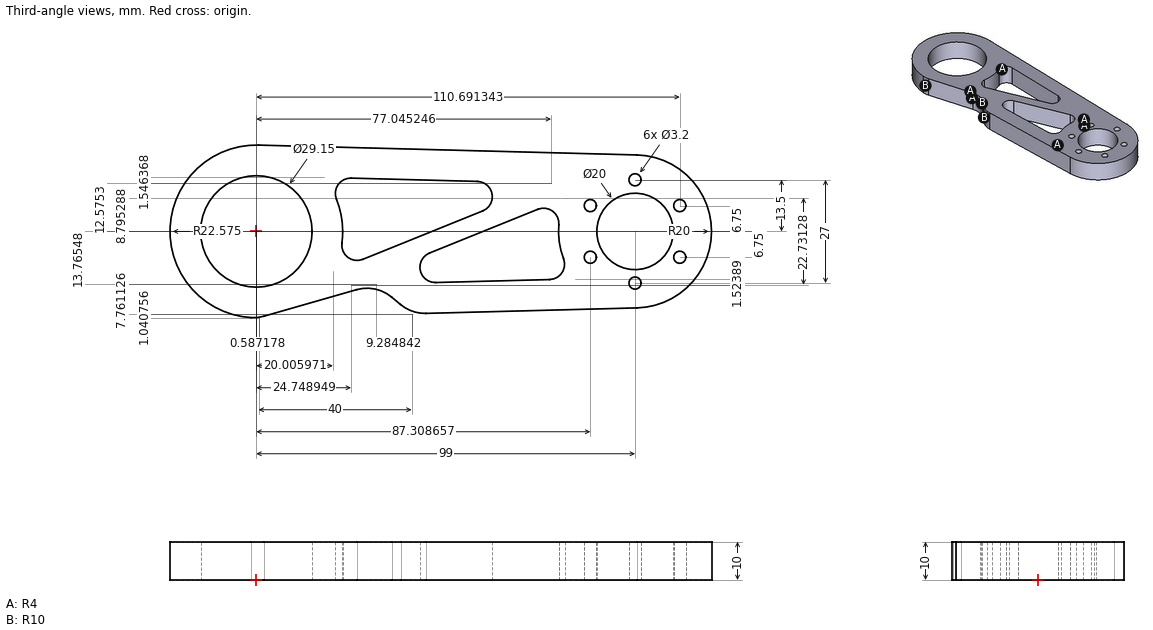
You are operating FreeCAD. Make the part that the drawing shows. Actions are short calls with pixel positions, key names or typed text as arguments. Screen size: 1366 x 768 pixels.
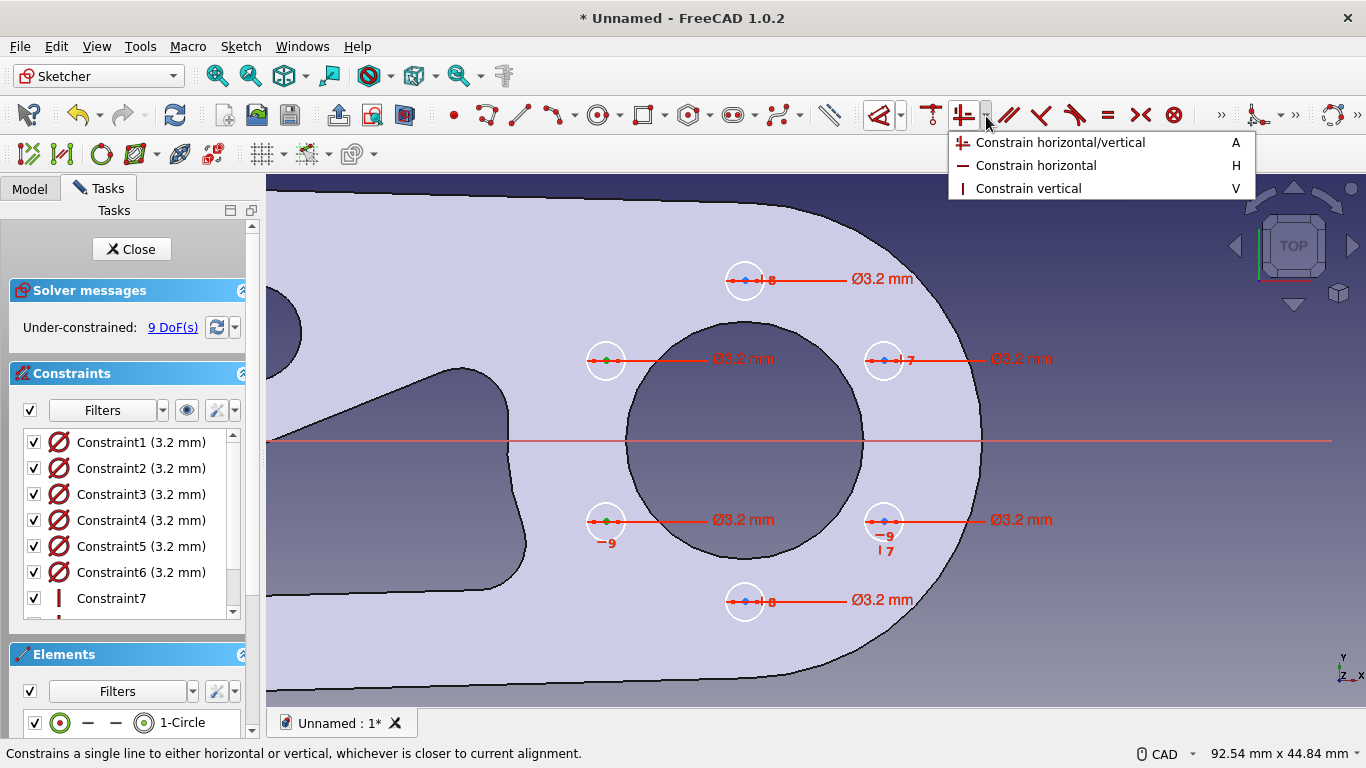
click(1102, 188)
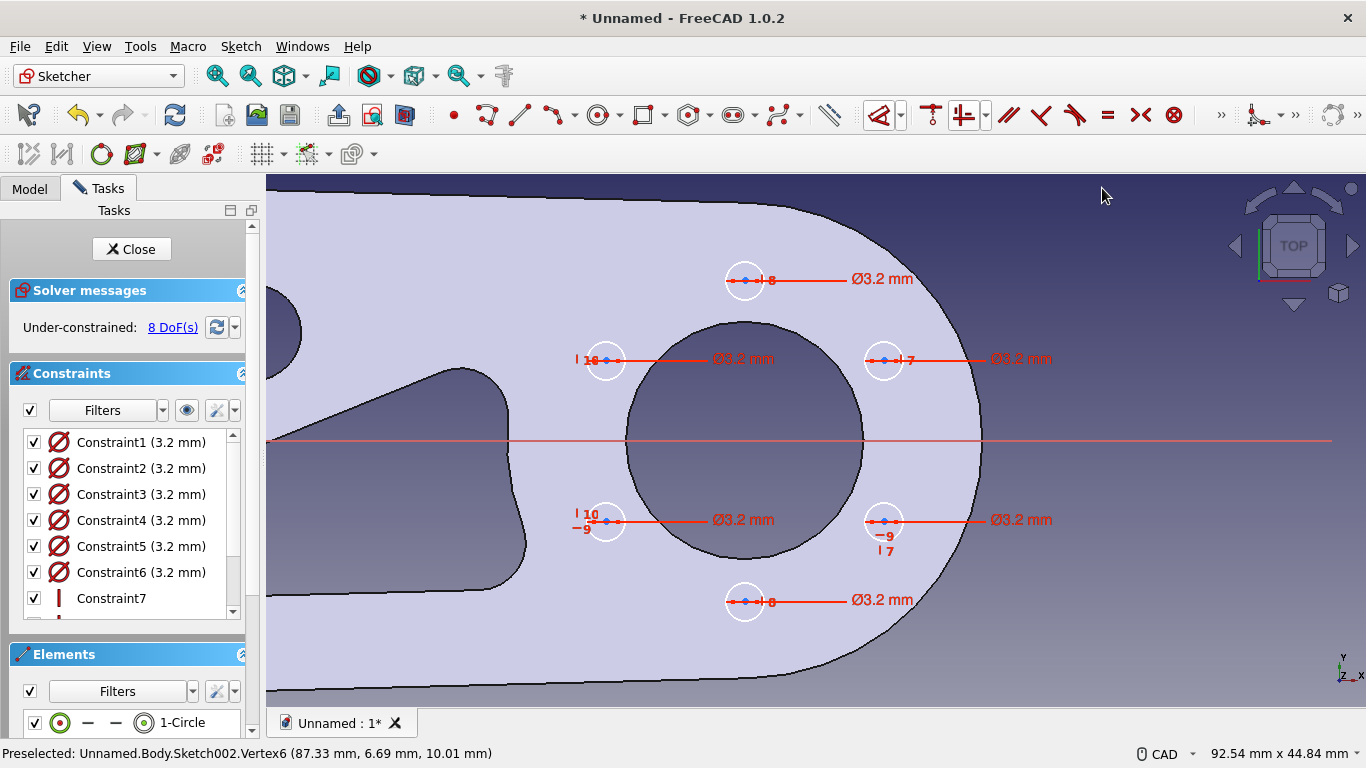
click(884, 361)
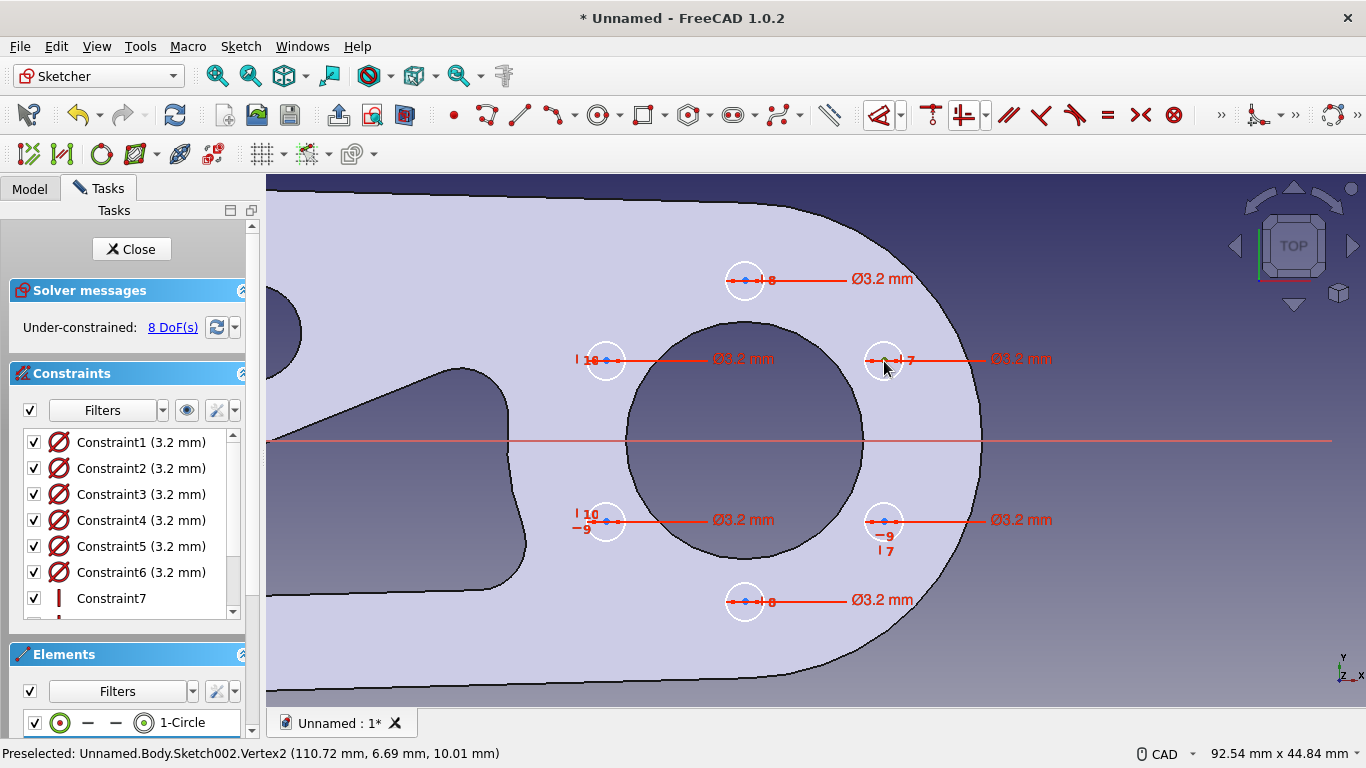
click(606, 361)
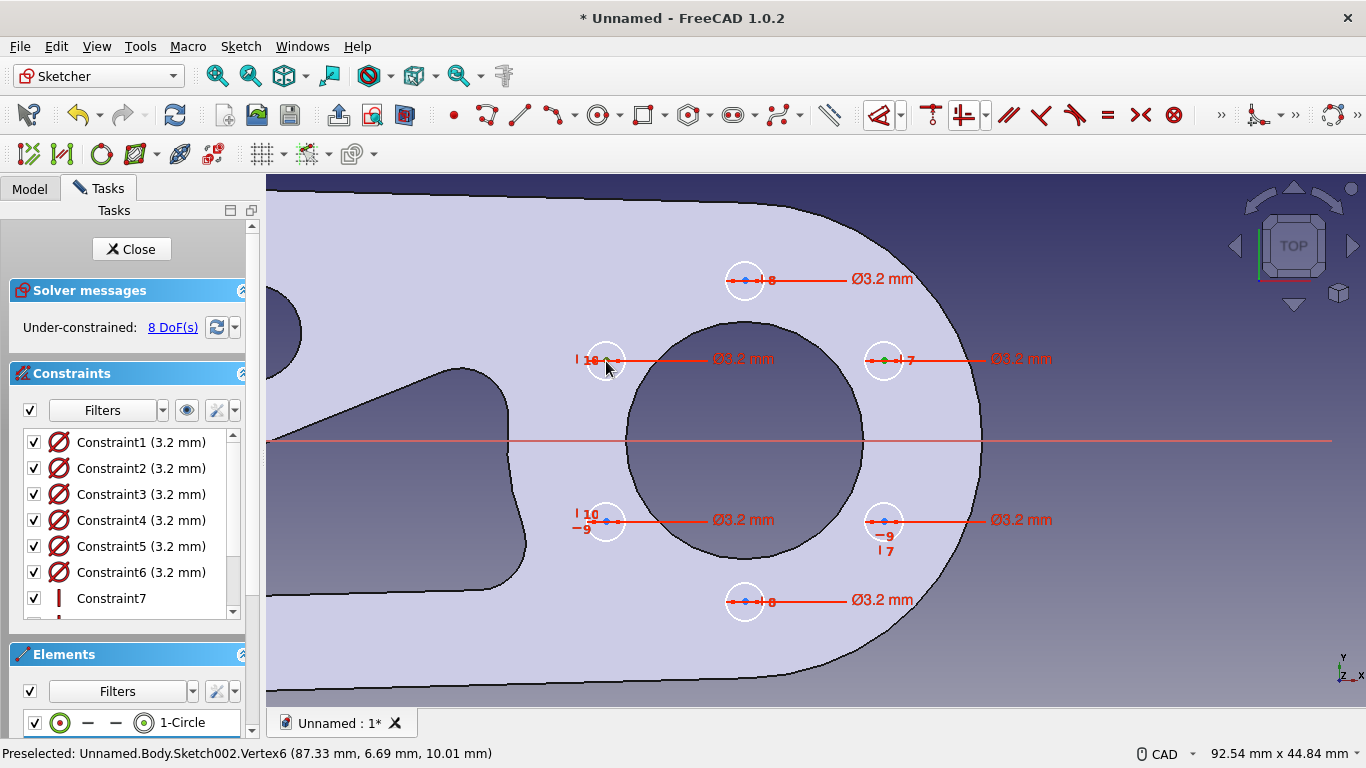
click(986, 116)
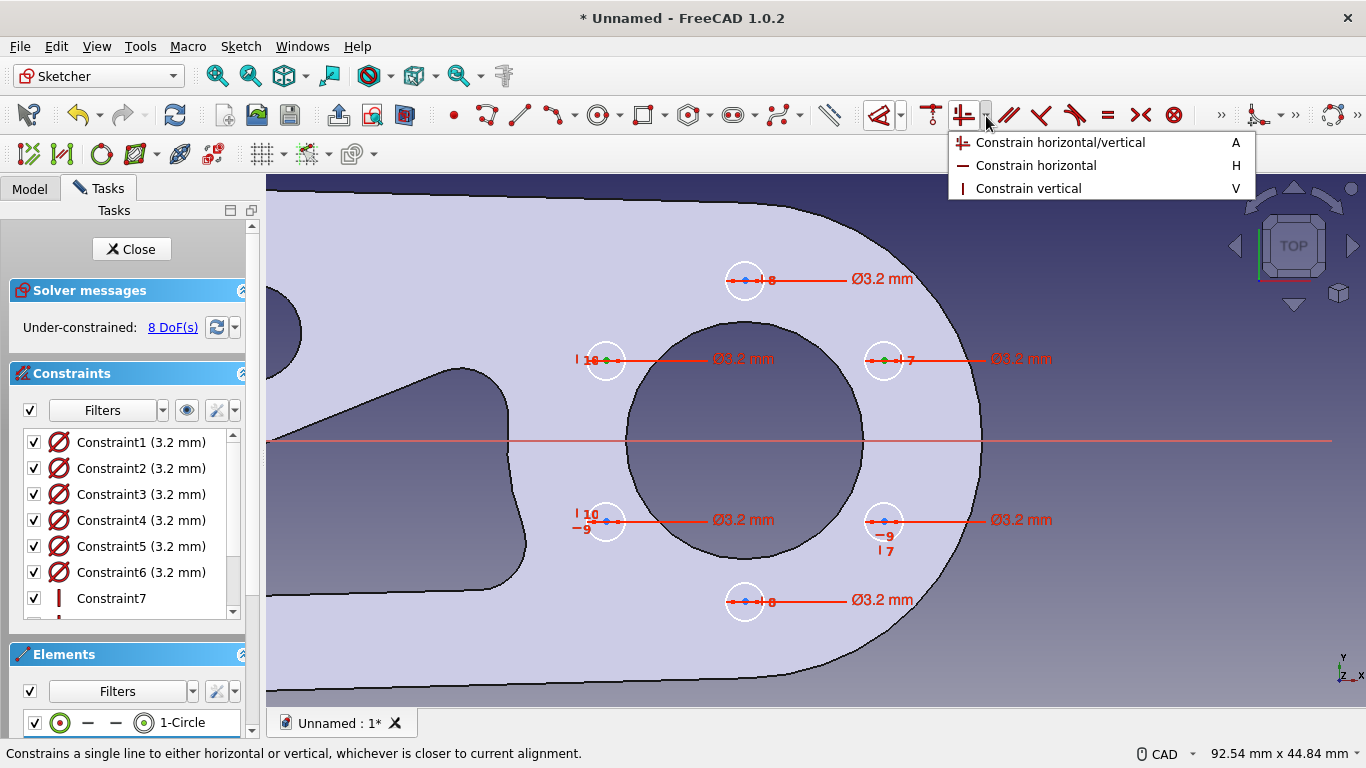
click(1102, 166)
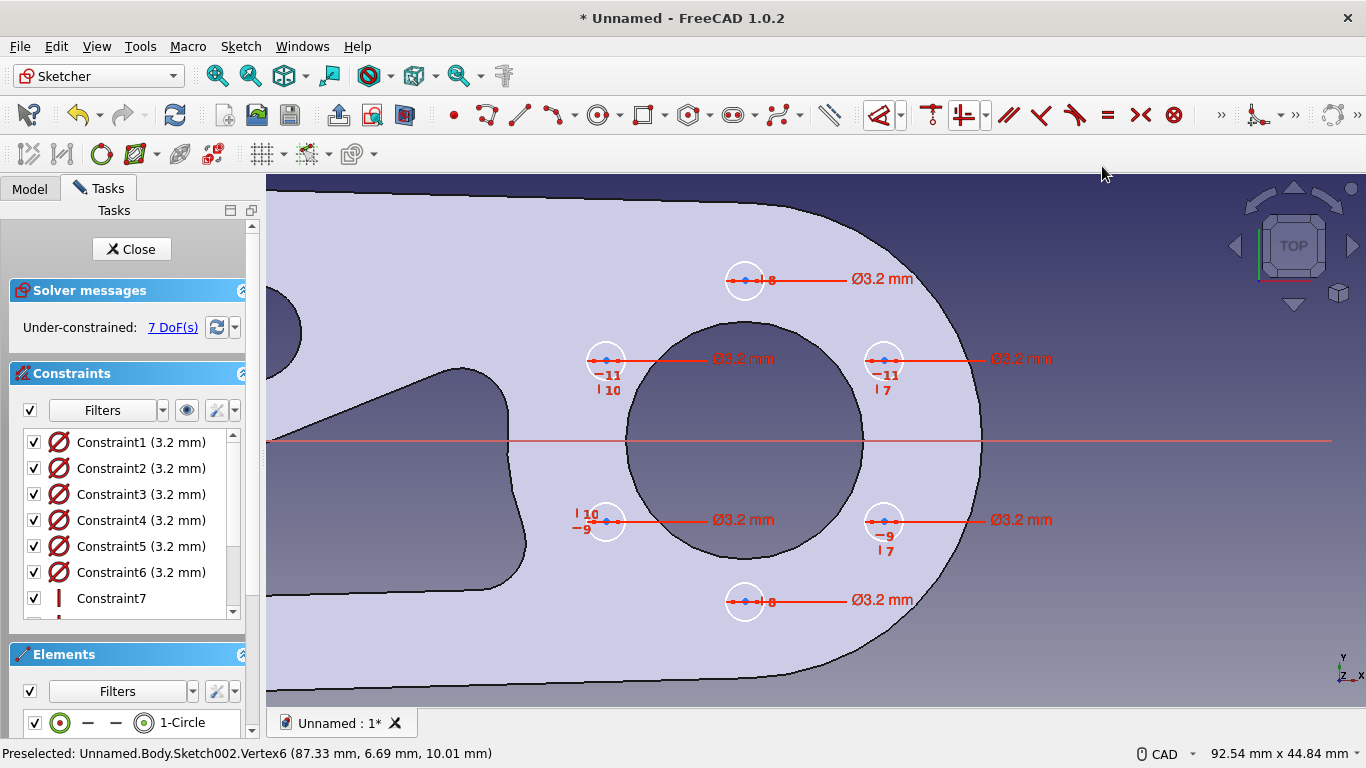
click(745, 281)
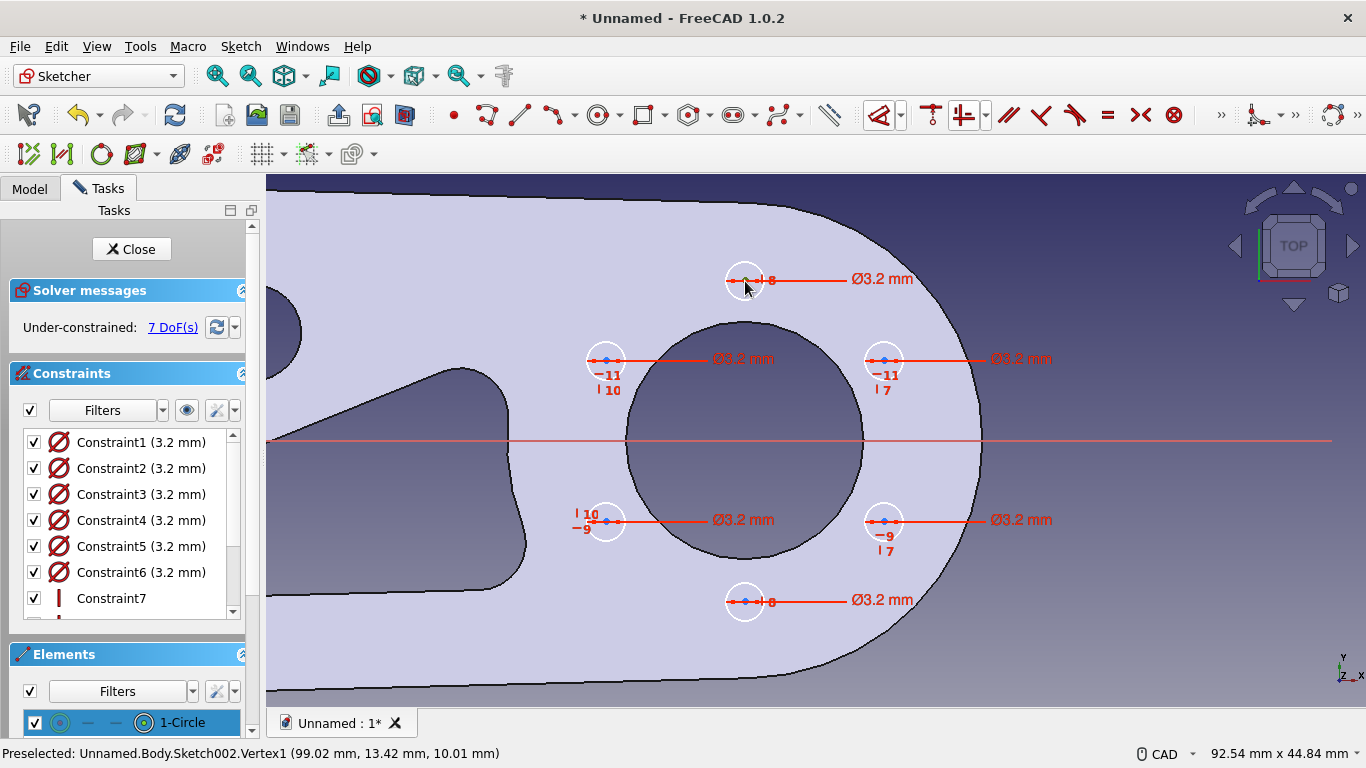
click(900, 116)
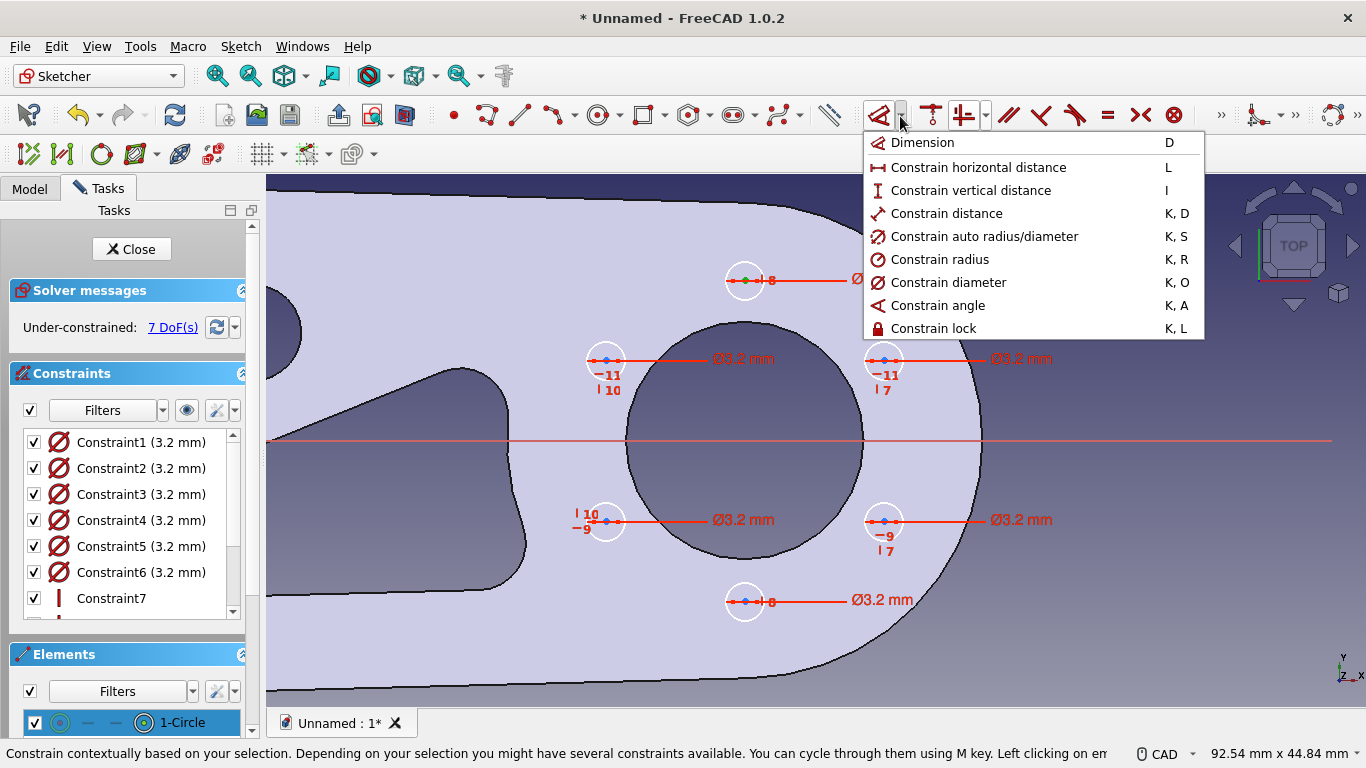
click(1034, 168)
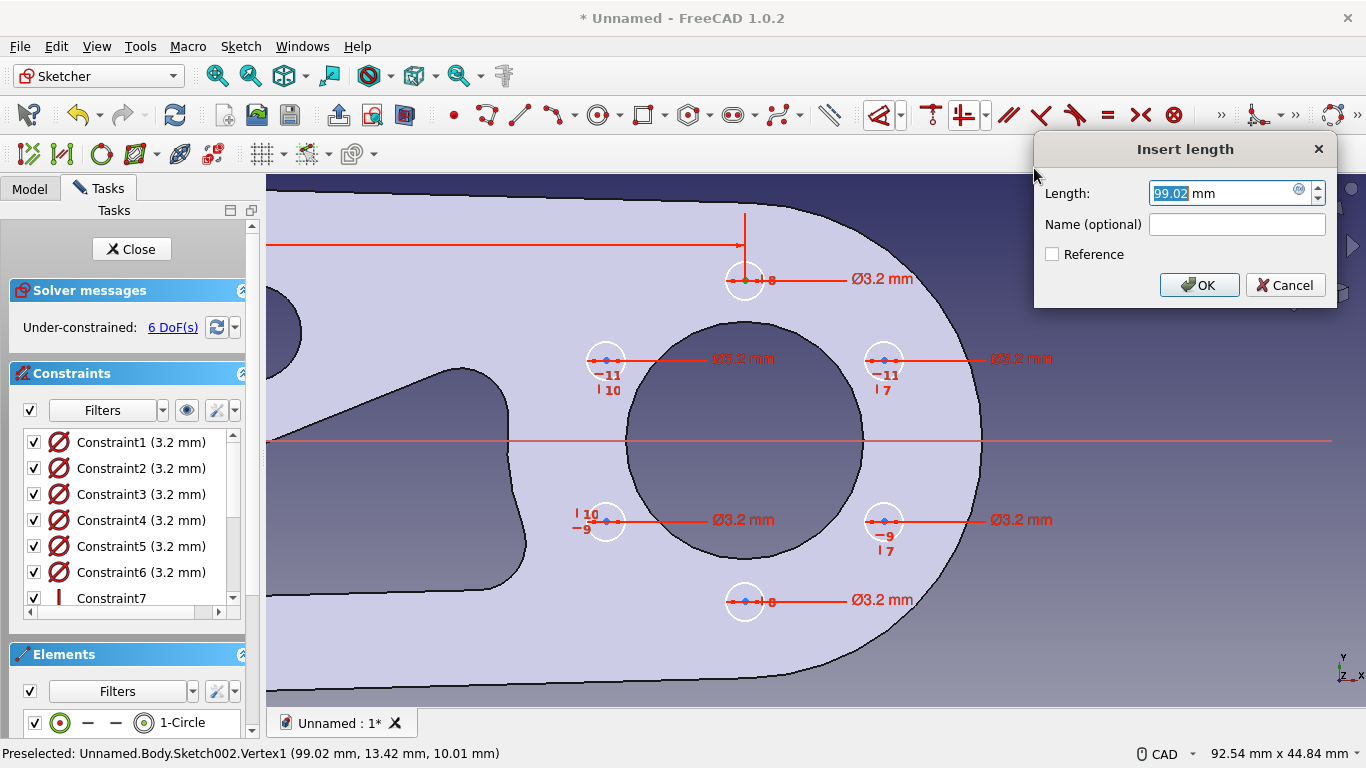
text(99)
key(Return)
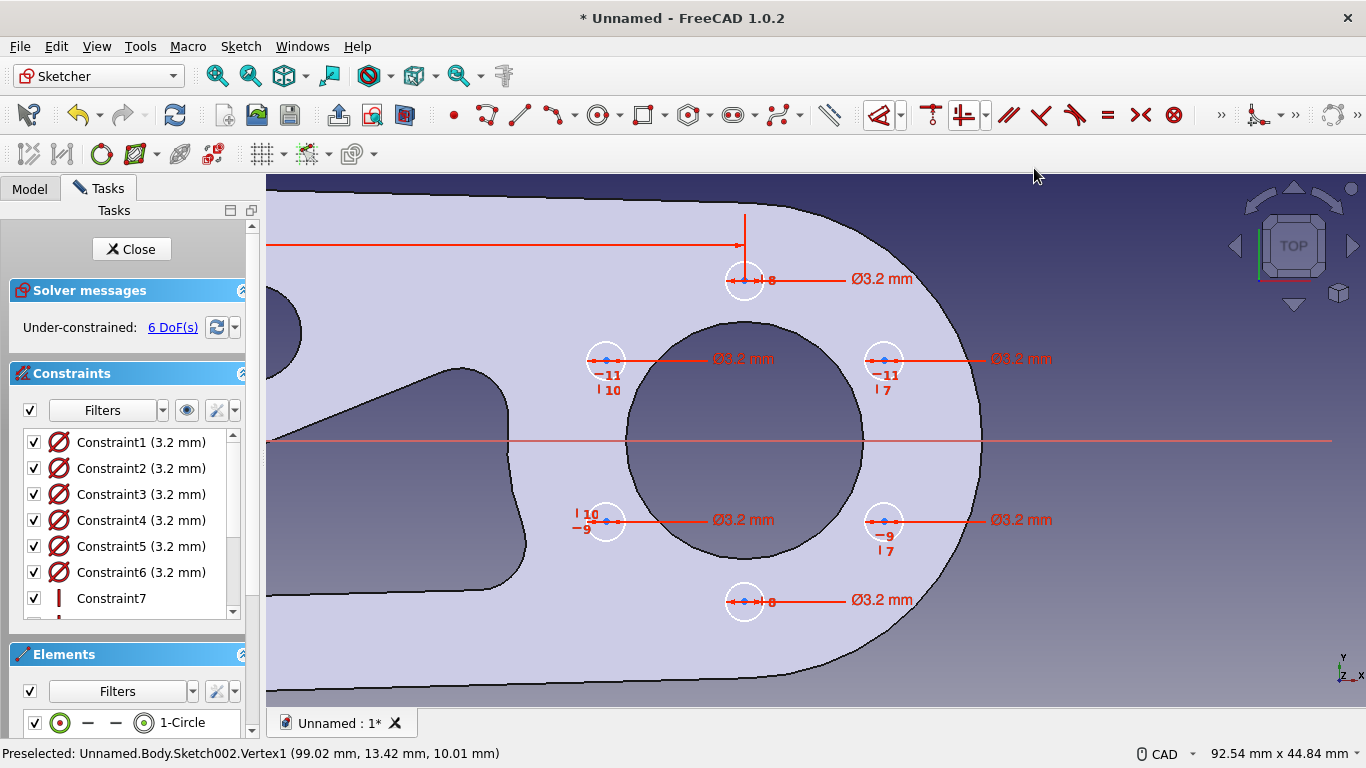
click(745, 281)